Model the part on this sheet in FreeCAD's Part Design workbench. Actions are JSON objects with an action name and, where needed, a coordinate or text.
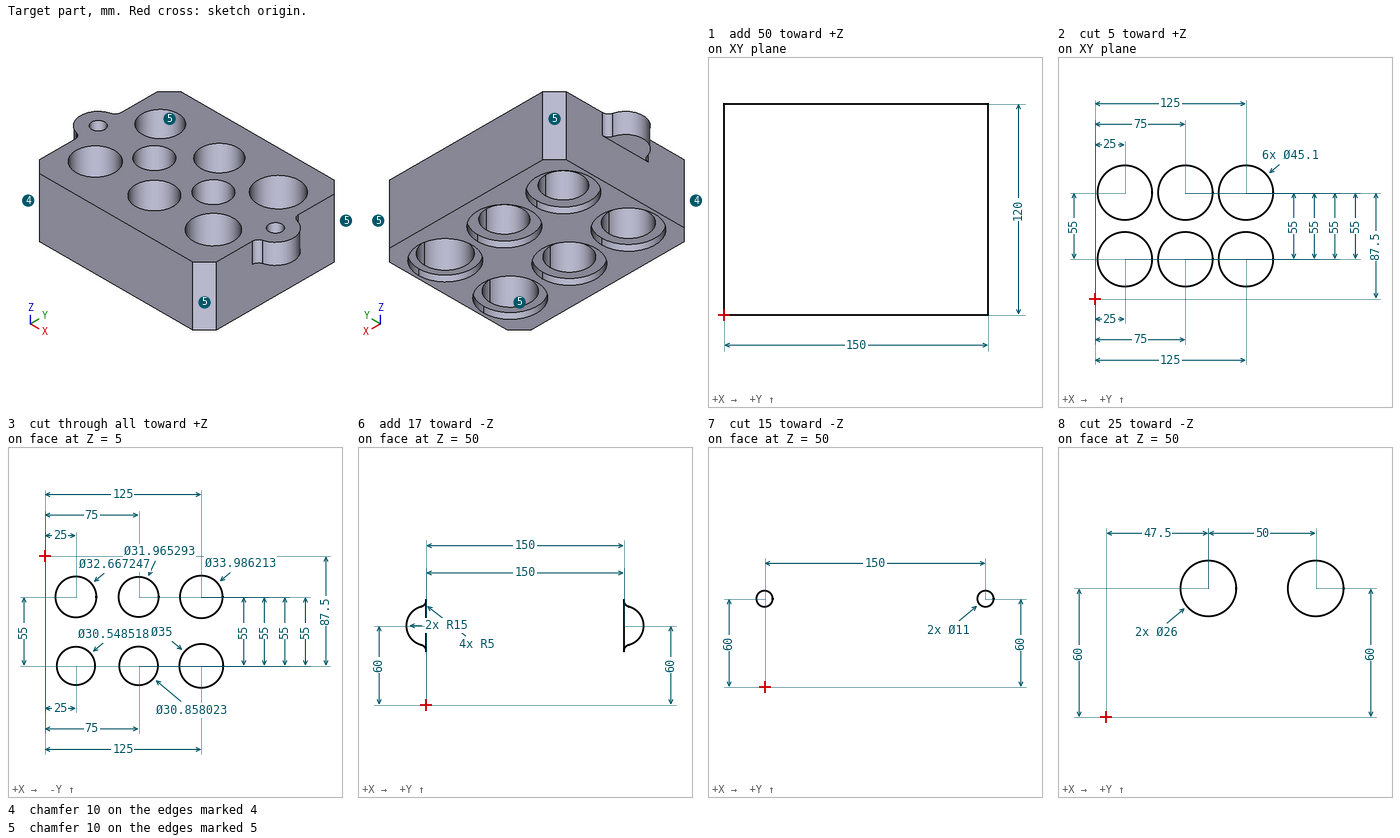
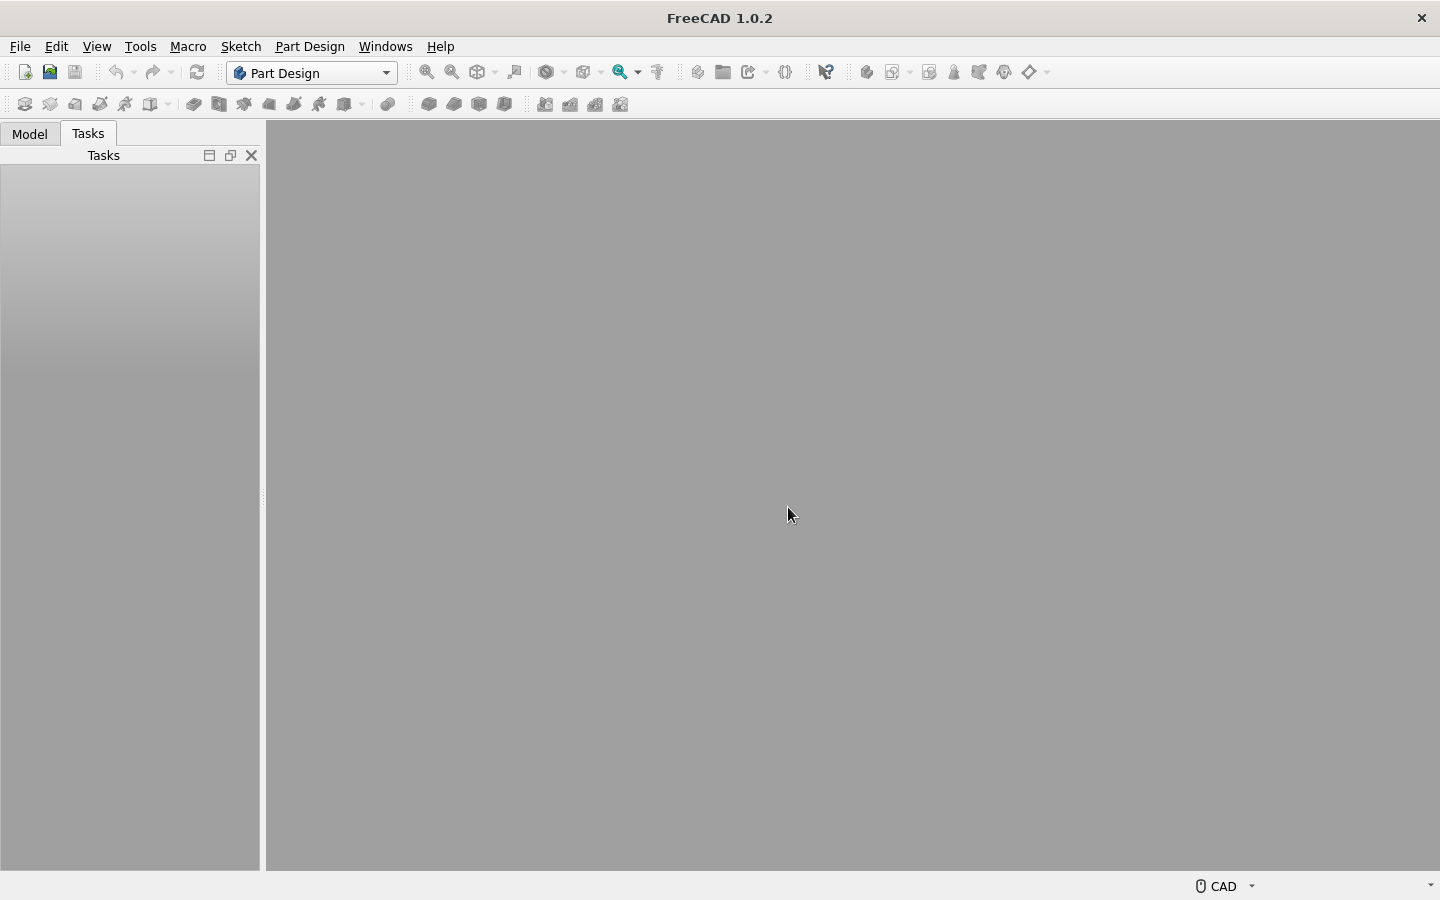
{"action": "left_click", "coordinate": [25, 72]}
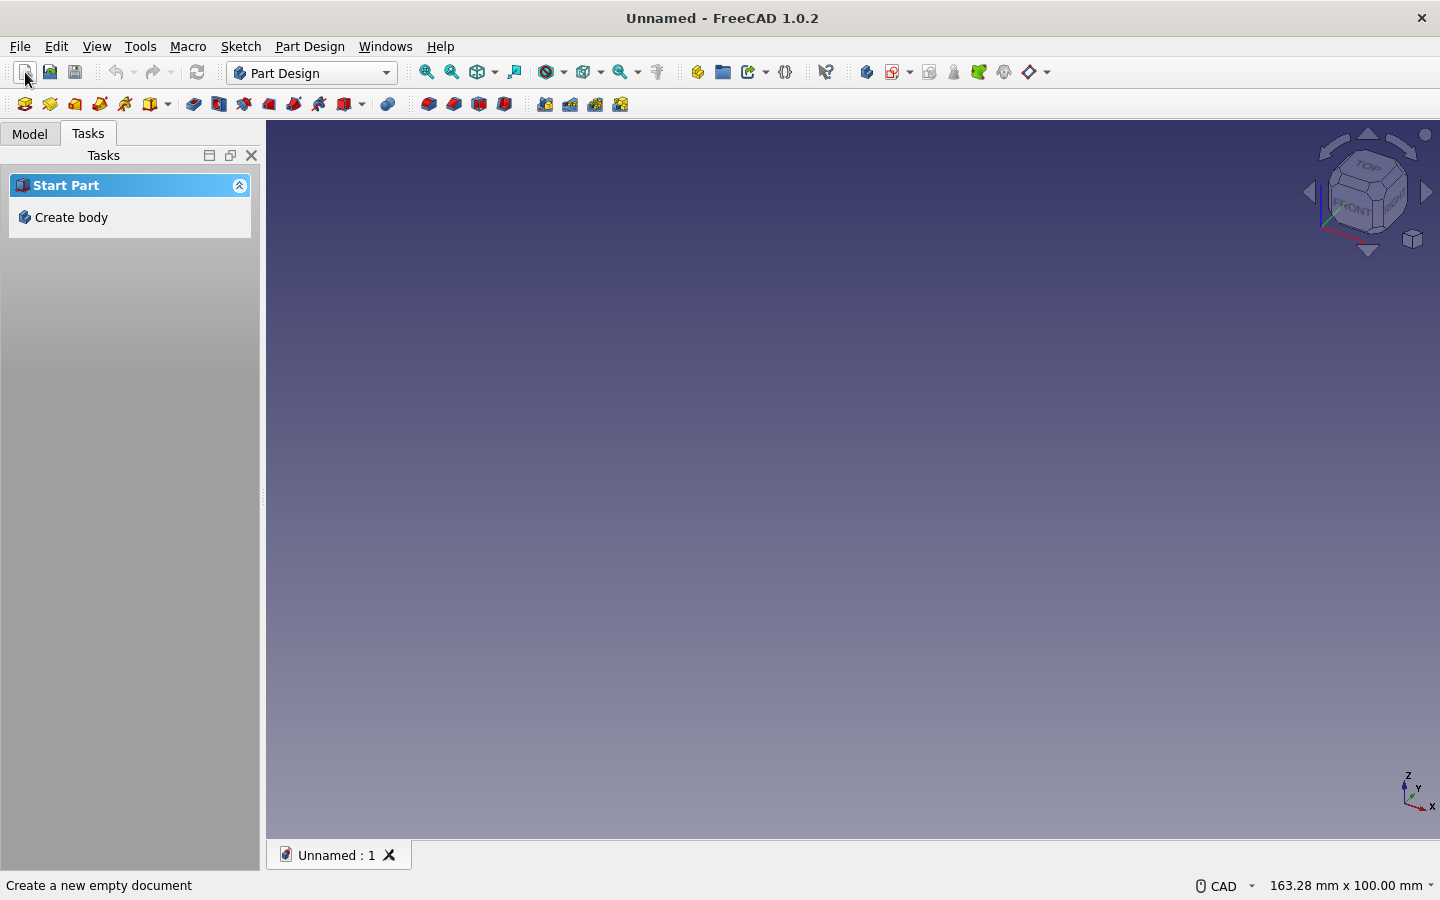
{"action": "left_click", "coordinate": [892, 72]}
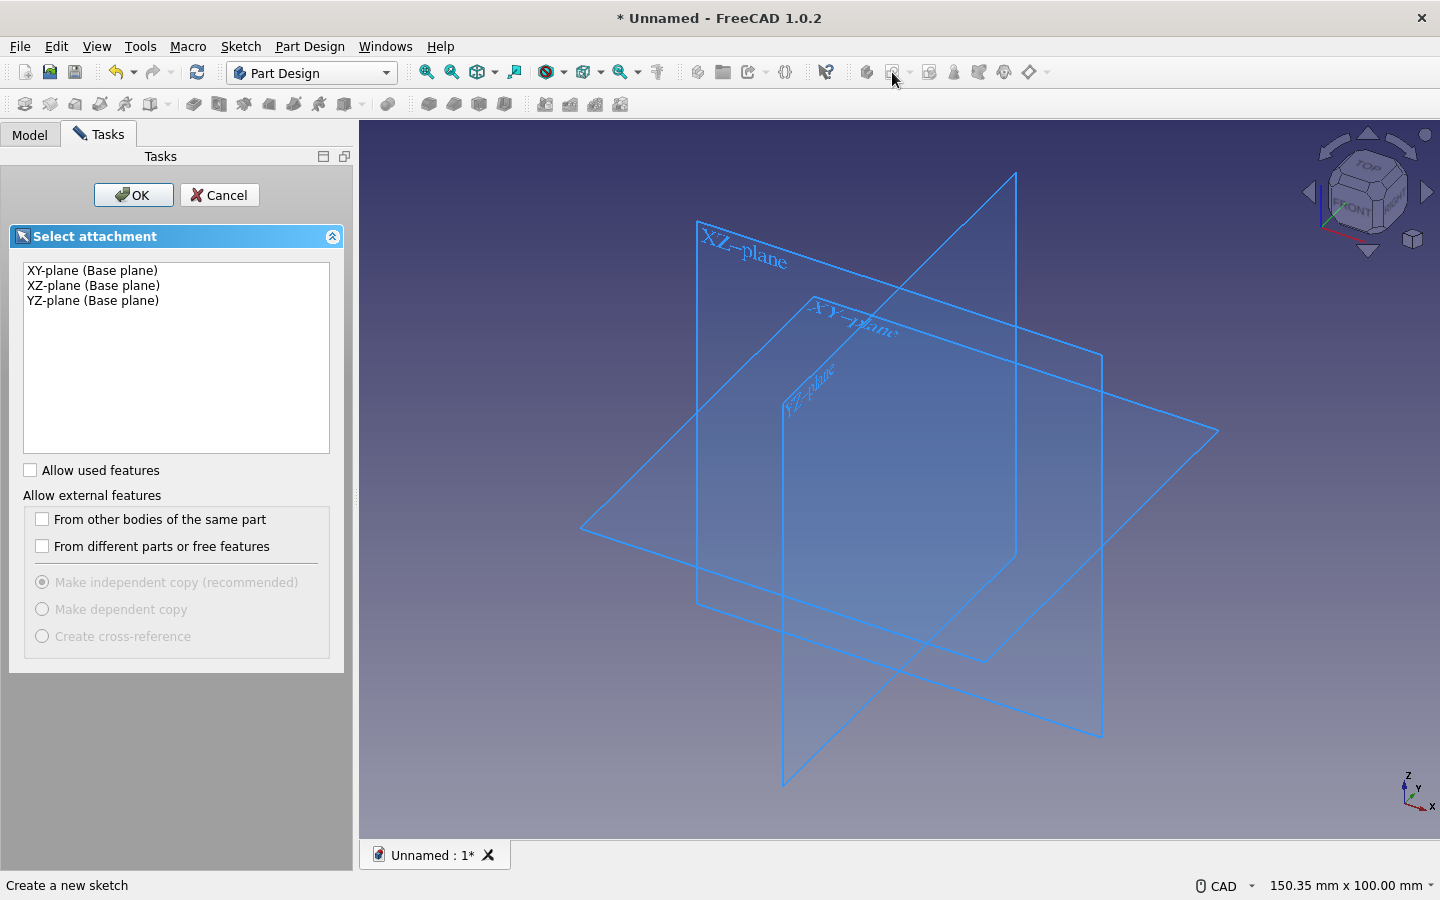
{"action": "left_click", "coordinate": [84, 270]}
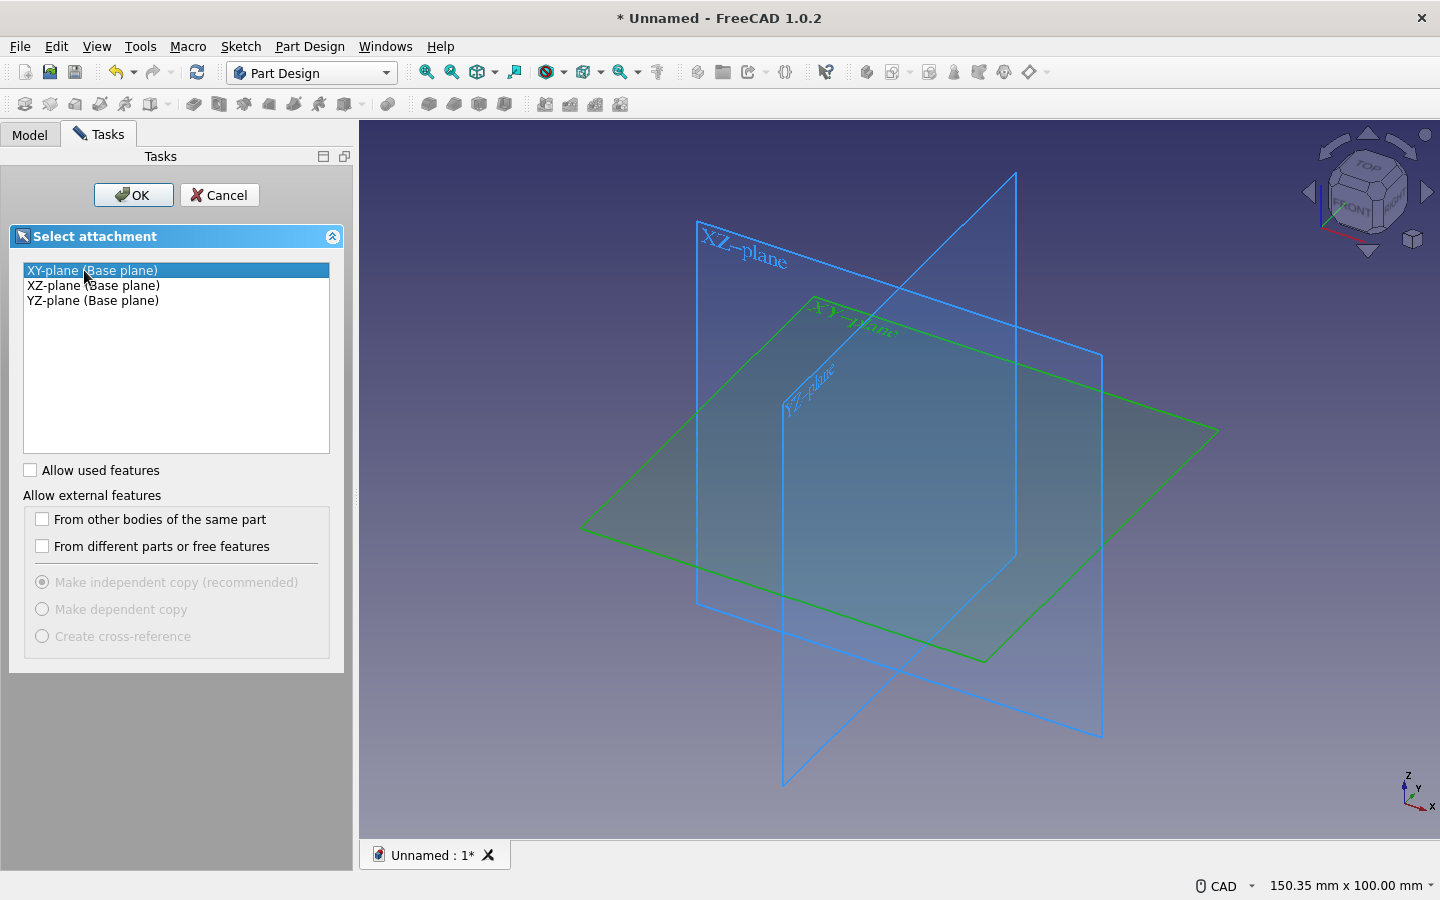
{"action": "left_click", "coordinate": [134, 195]}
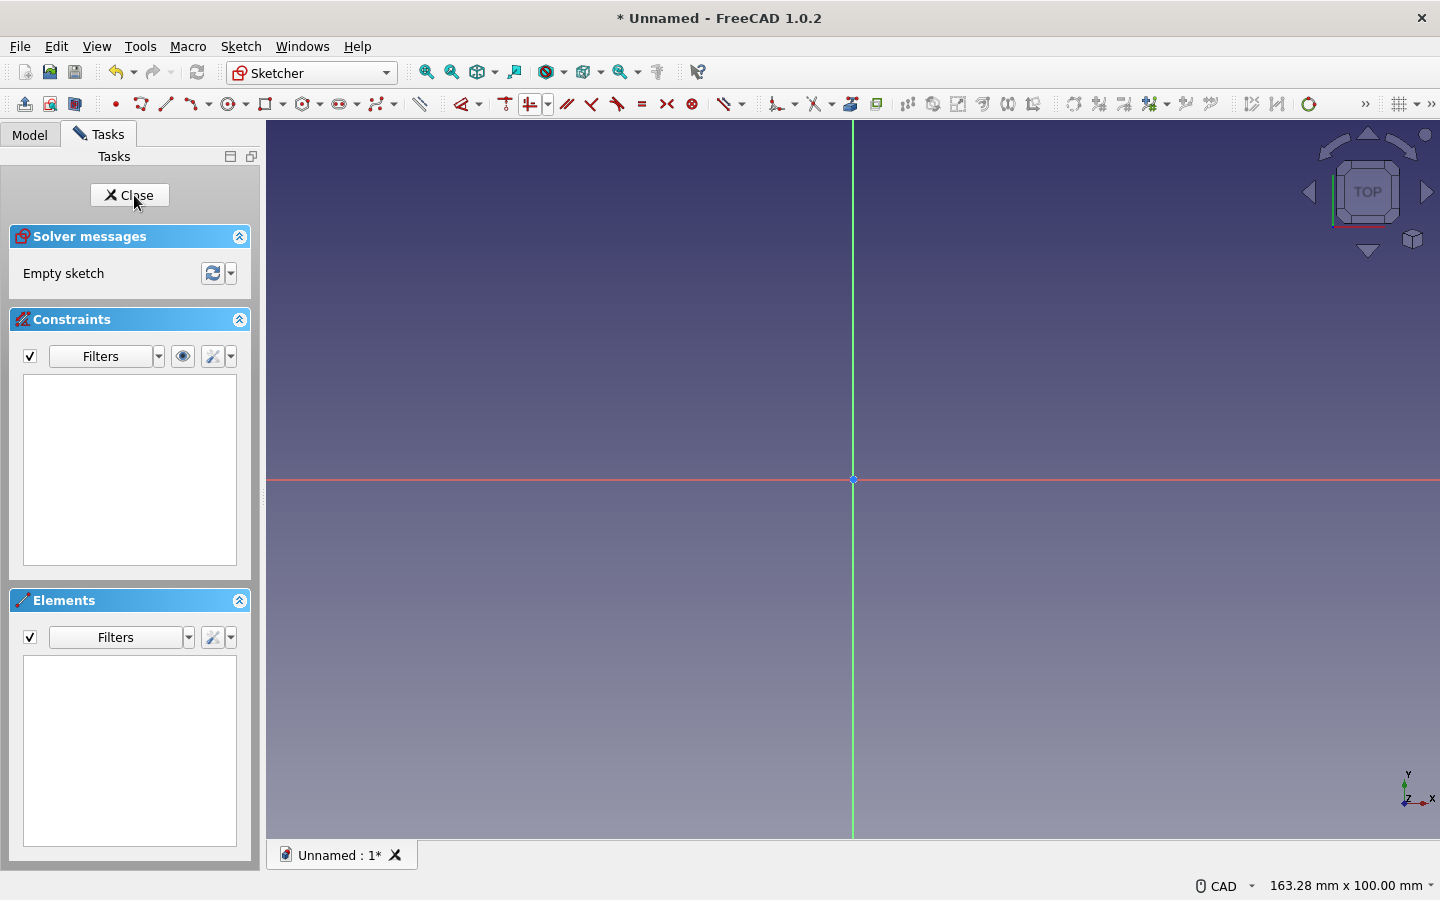
{"action": "scroll", "coordinate": [294, 811], "scroll_direction": "down", "scroll_amount": 4}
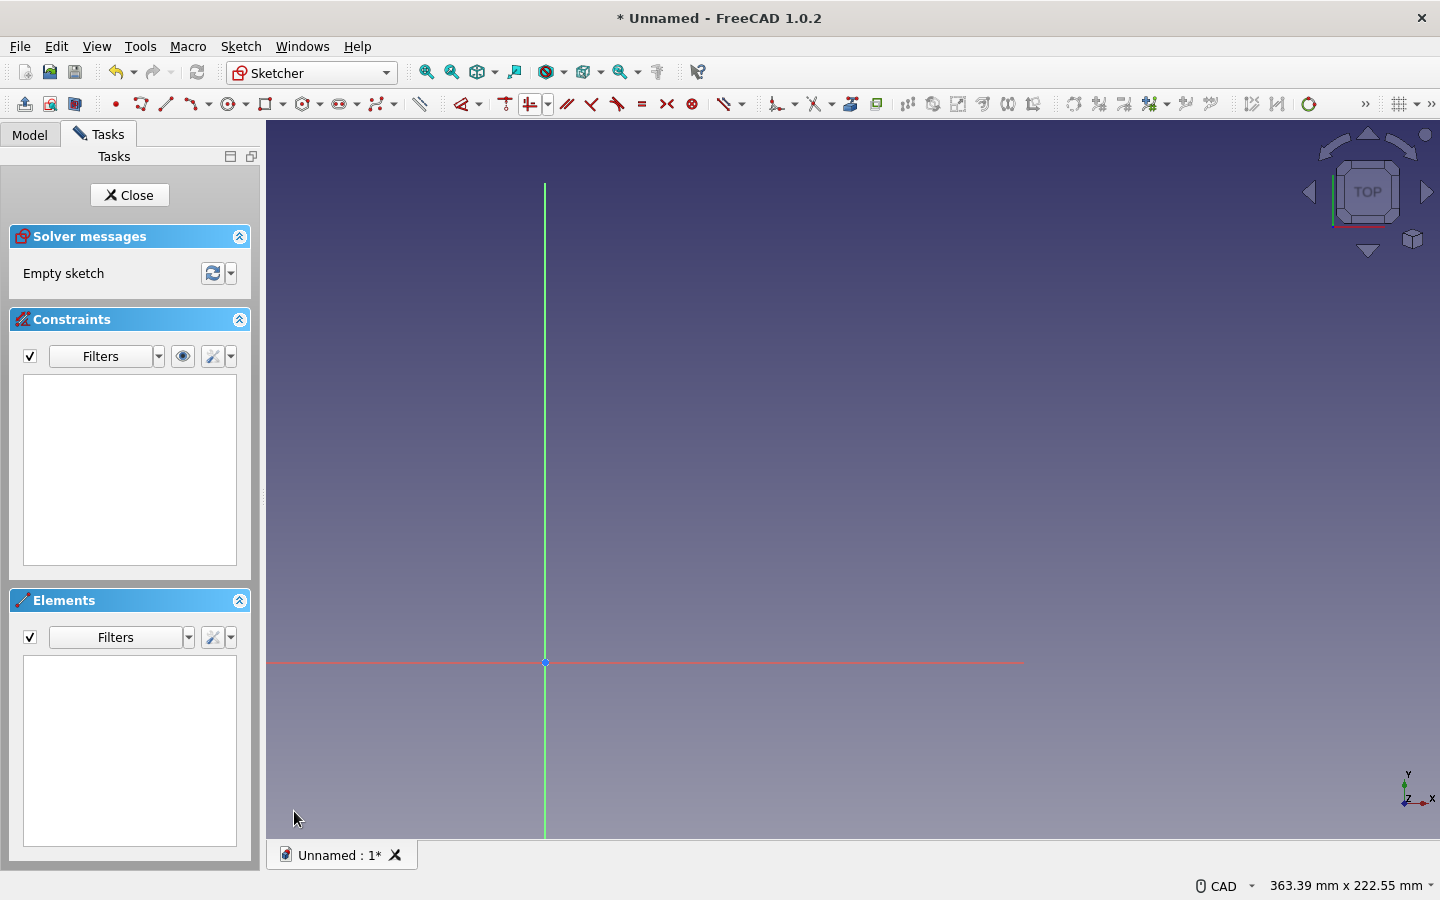
{"action": "left_click", "coordinate": [264, 104]}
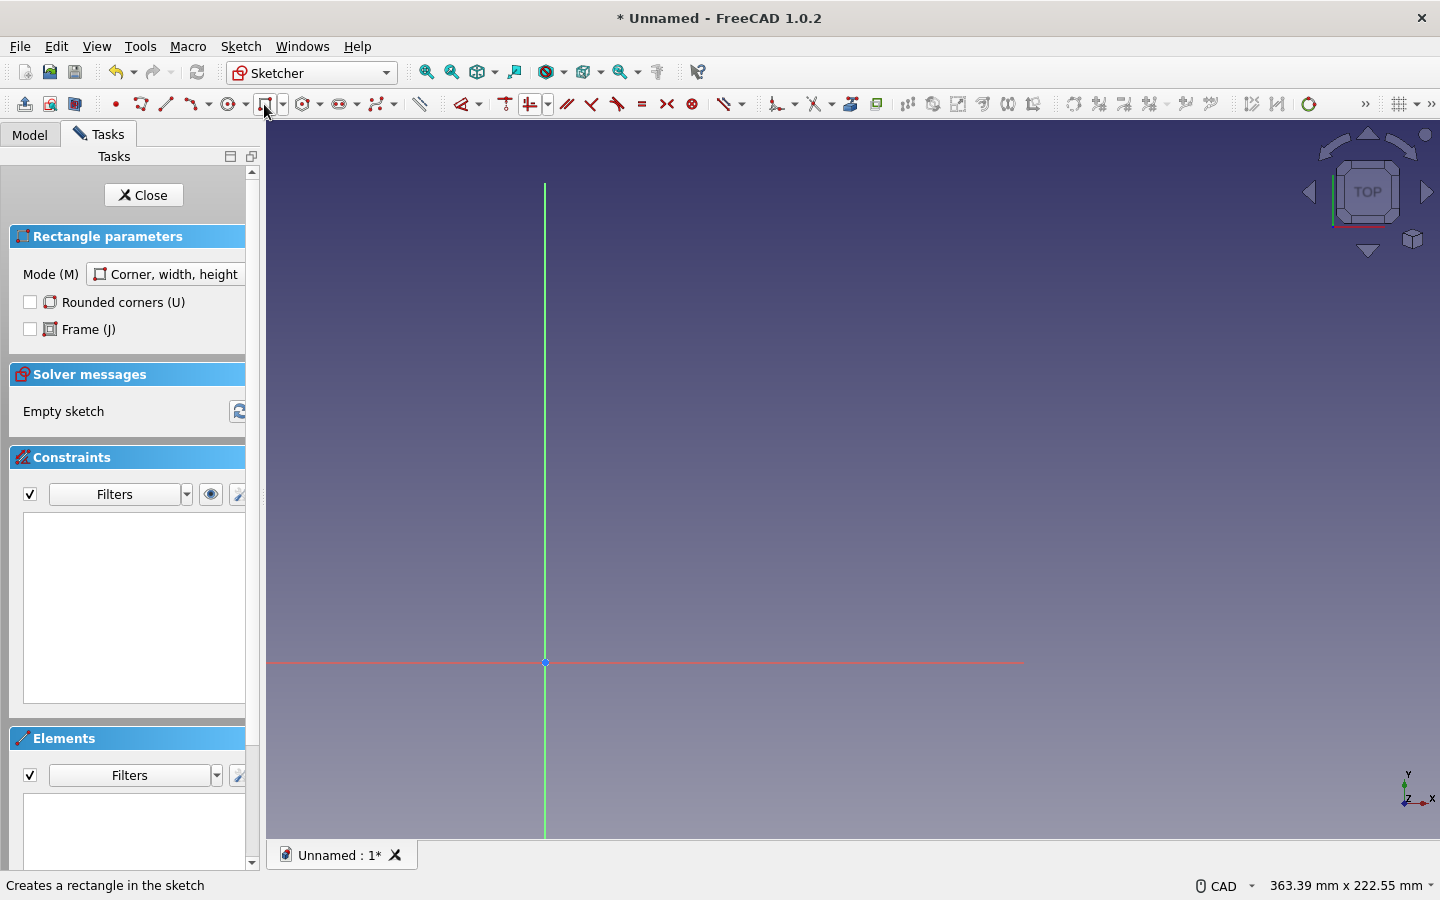
{"action": "left_click", "coordinate": [545, 663]}
{"action": "left_click", "coordinate": [1030, 275]}
{"action": "key", "text": "Escape"}